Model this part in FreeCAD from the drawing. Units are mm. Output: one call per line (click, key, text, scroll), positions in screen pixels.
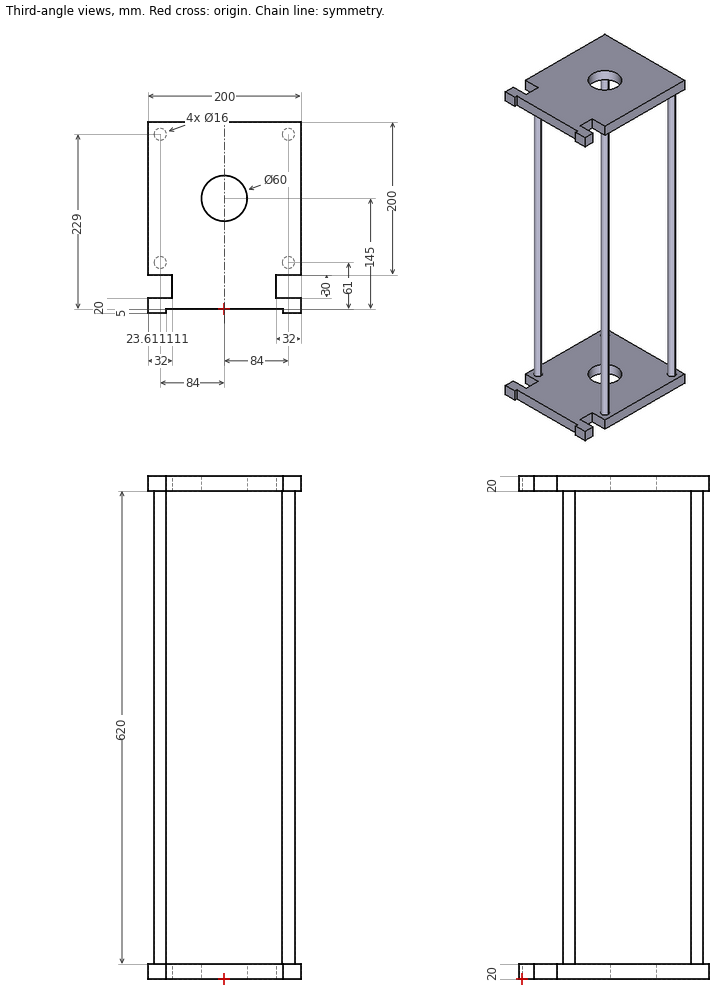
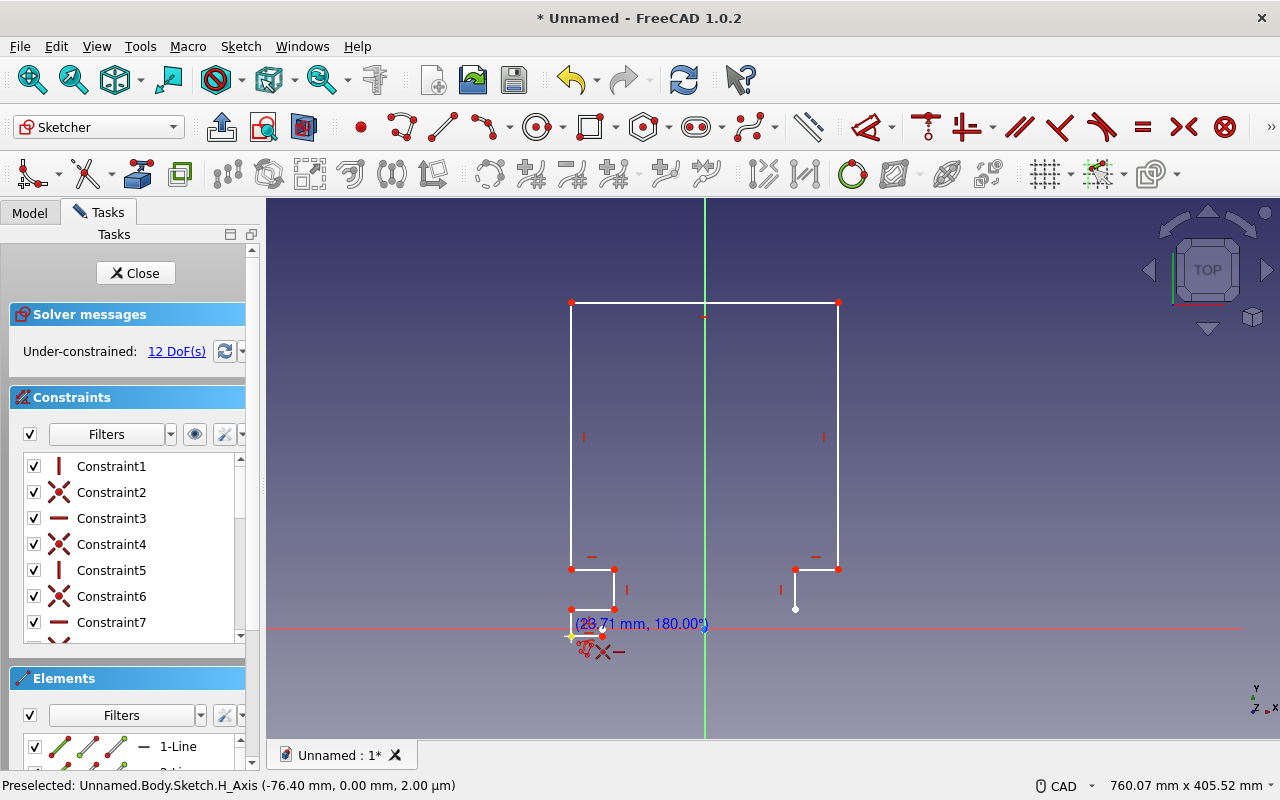
click(807, 620)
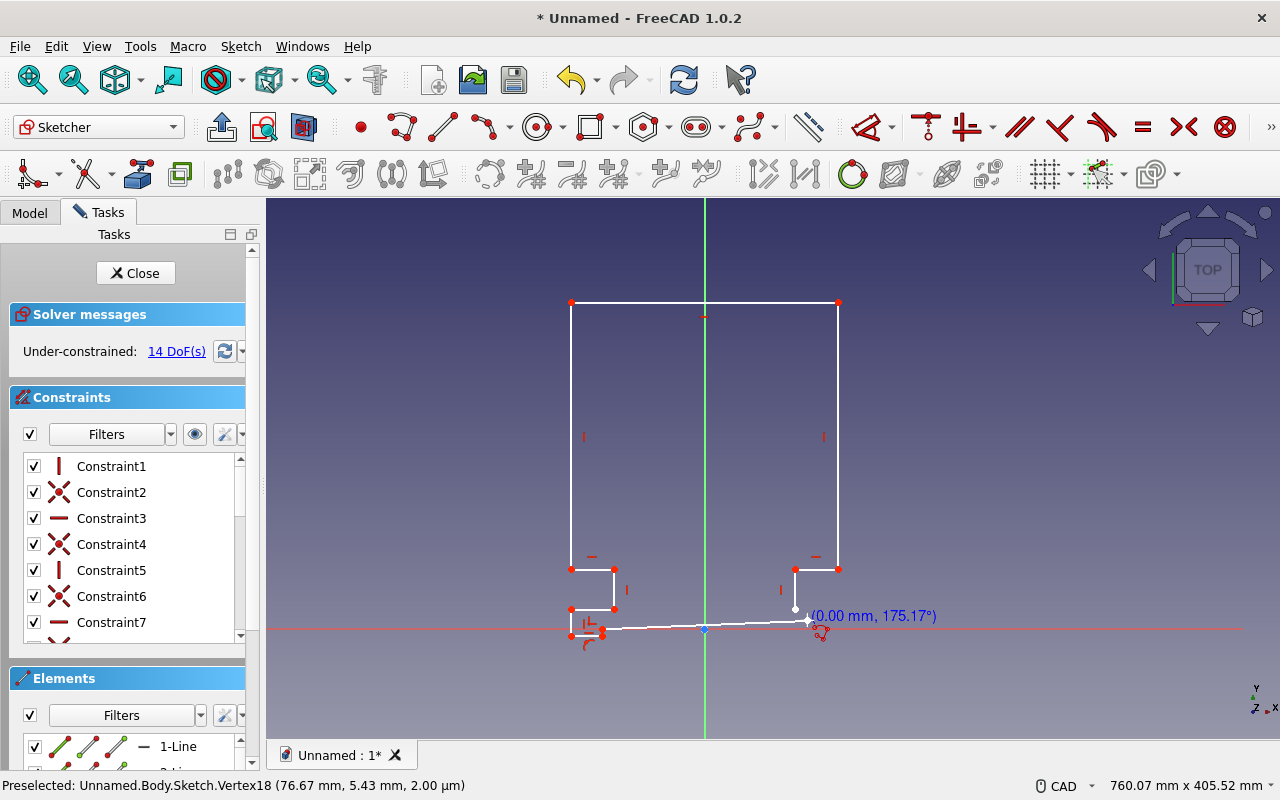
scroll(807, 636, up, 5)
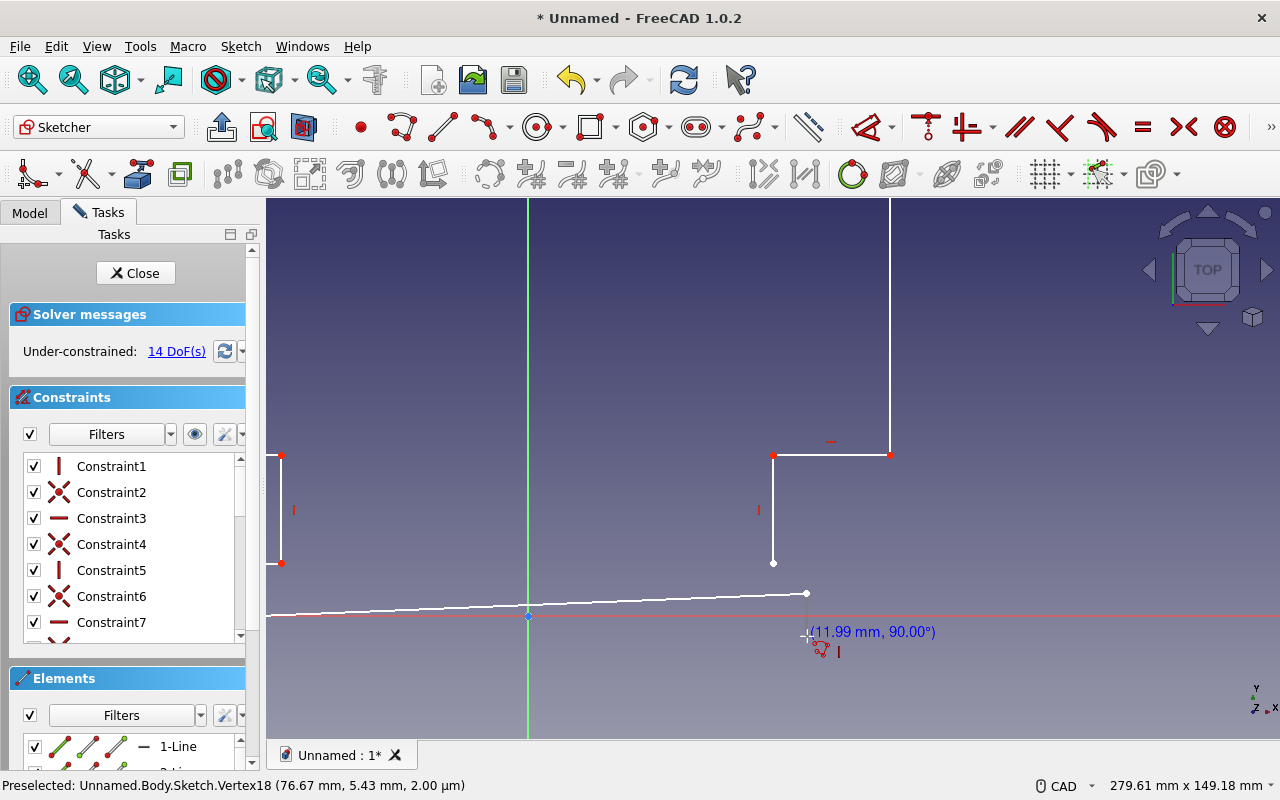
click(806, 634)
click(891, 634)
click(891, 562)
click(773, 564)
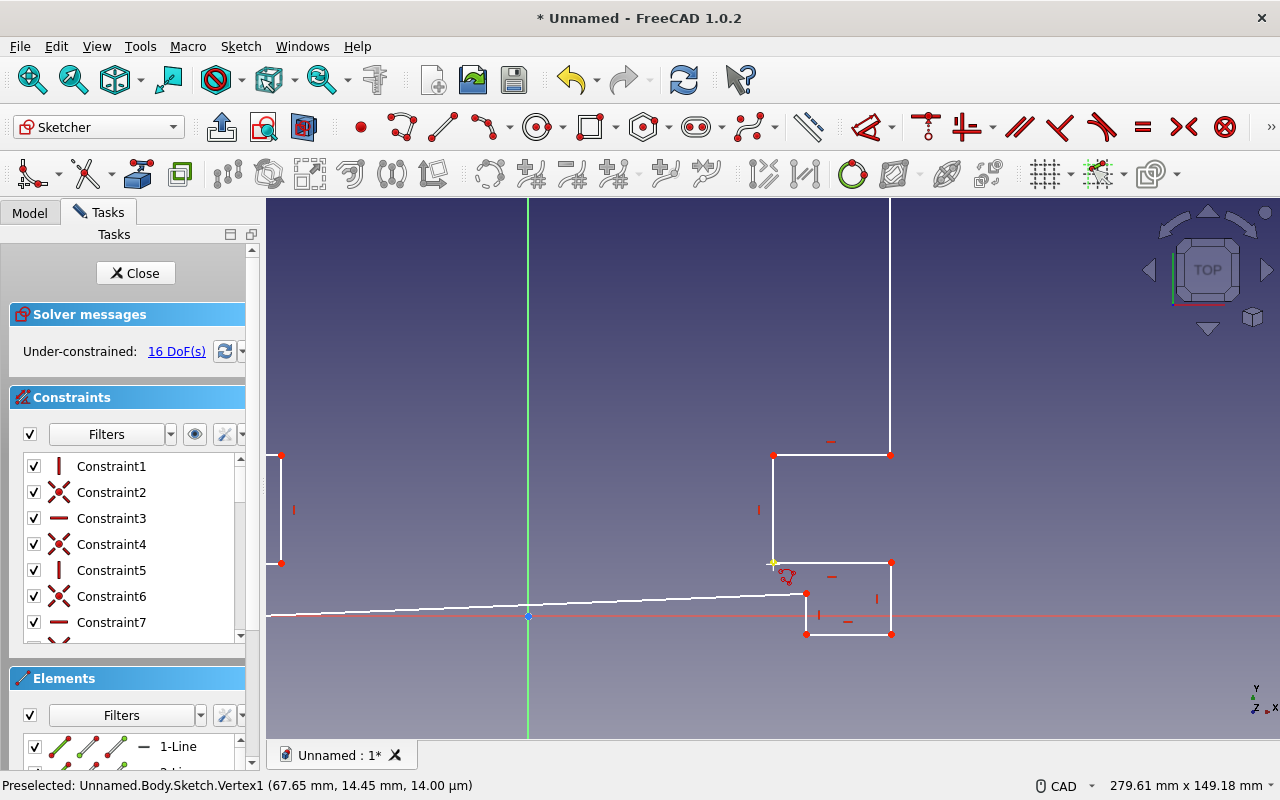
click(536, 128)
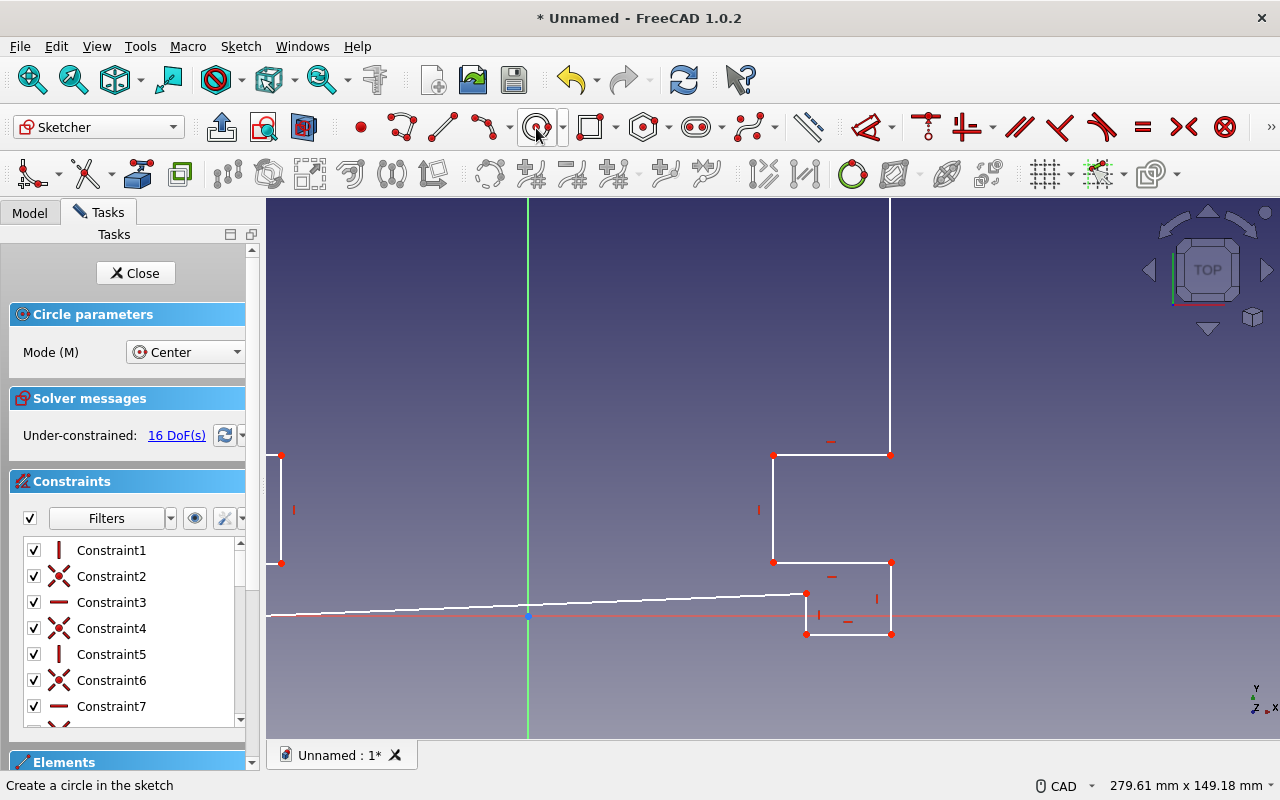
scroll(807, 636, down, 5)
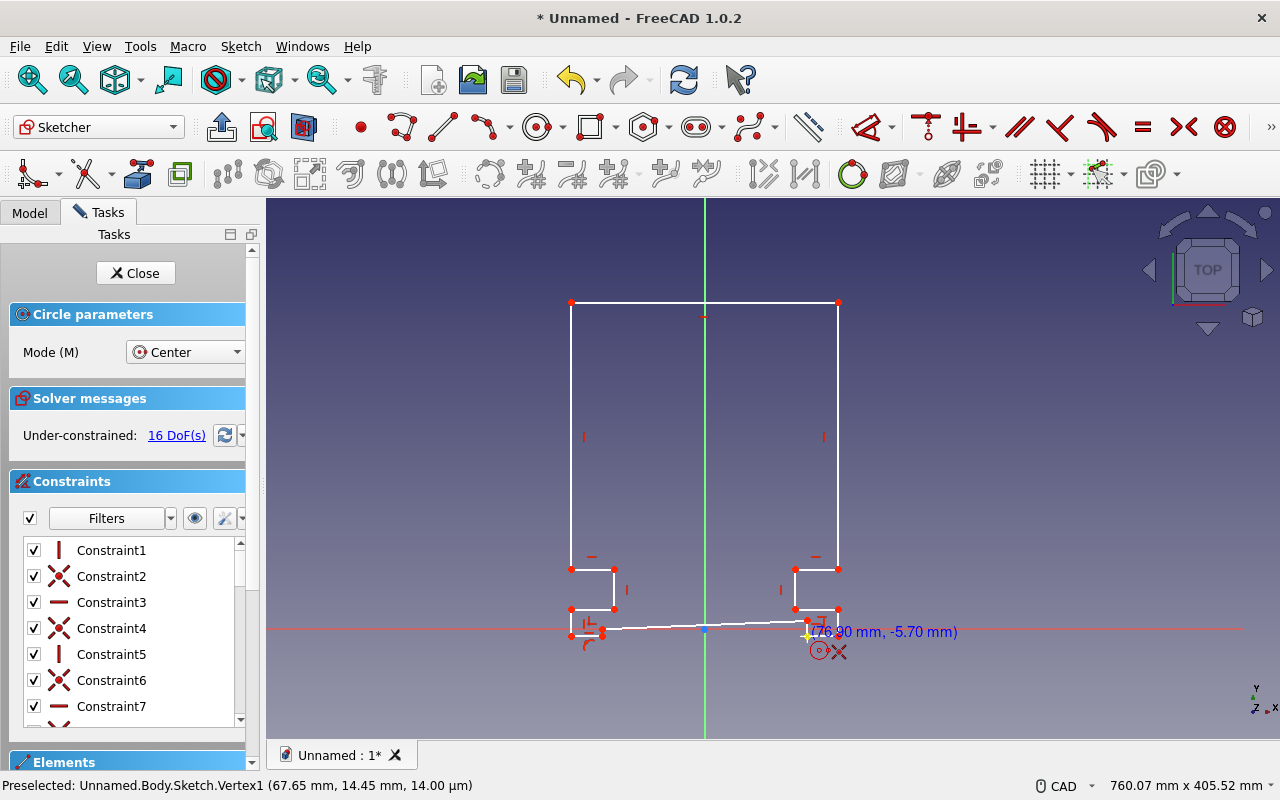
click(705, 436)
click(733, 408)
key(Escape)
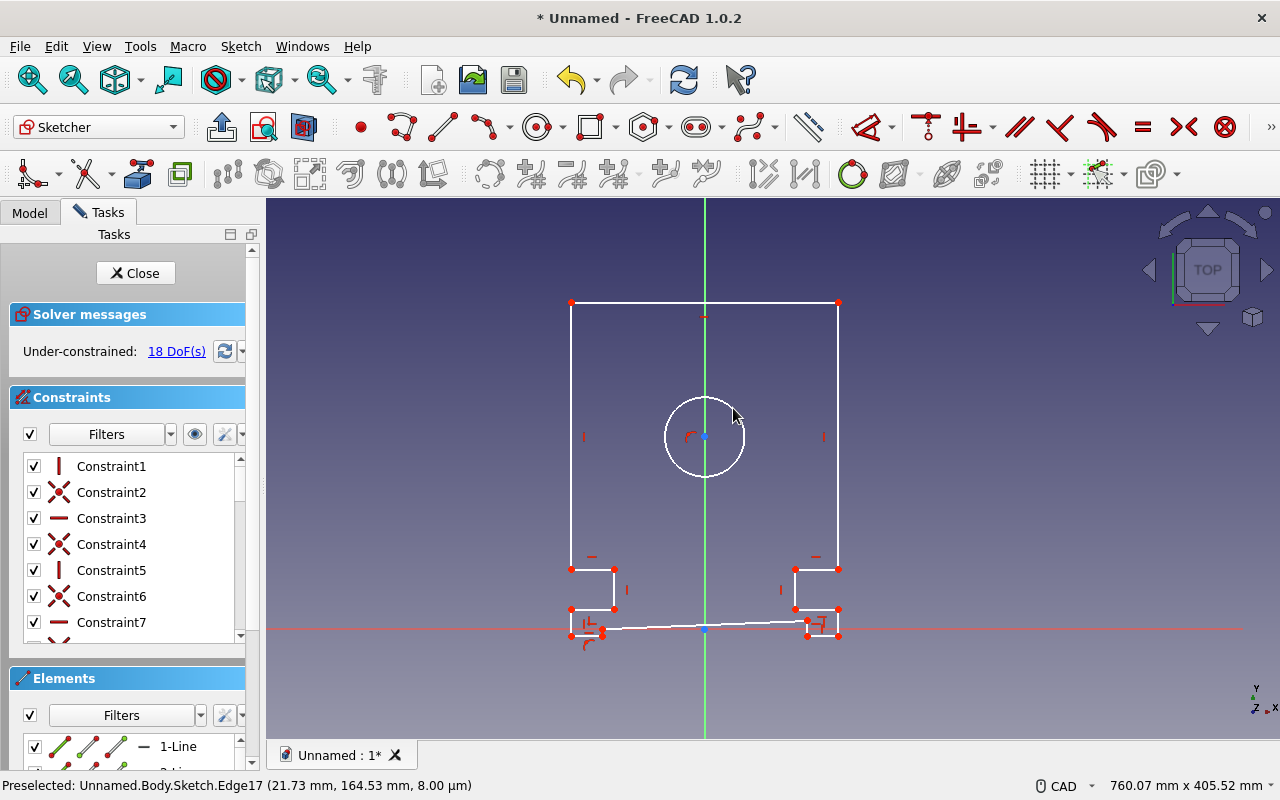
click(664, 627)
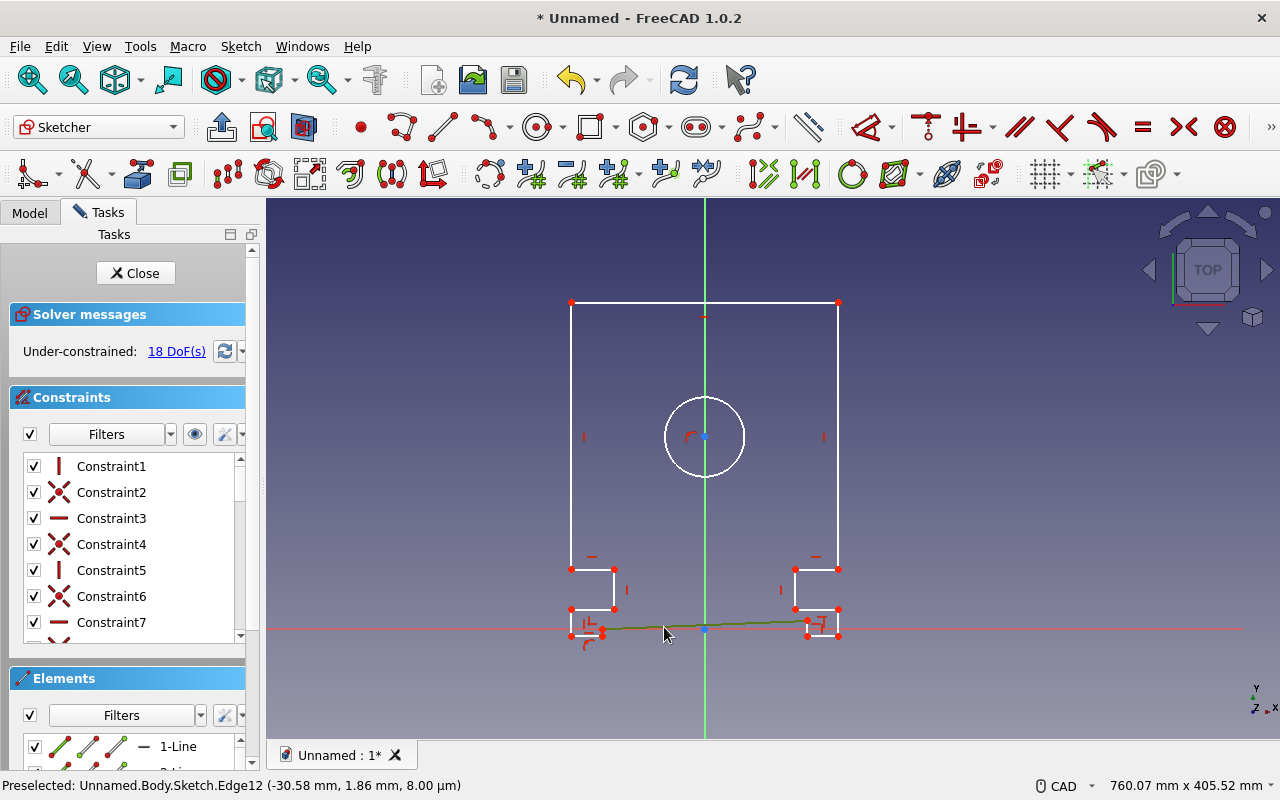
key(h)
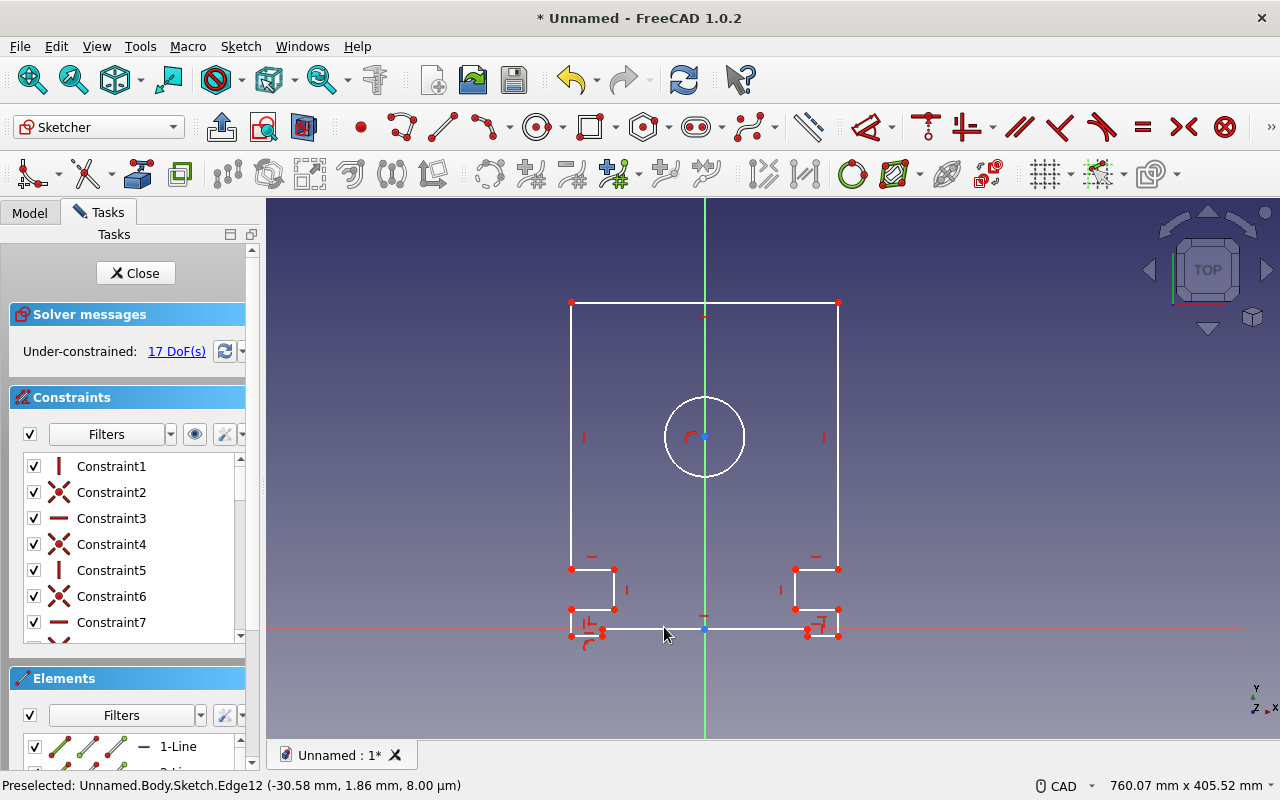
click(838, 570)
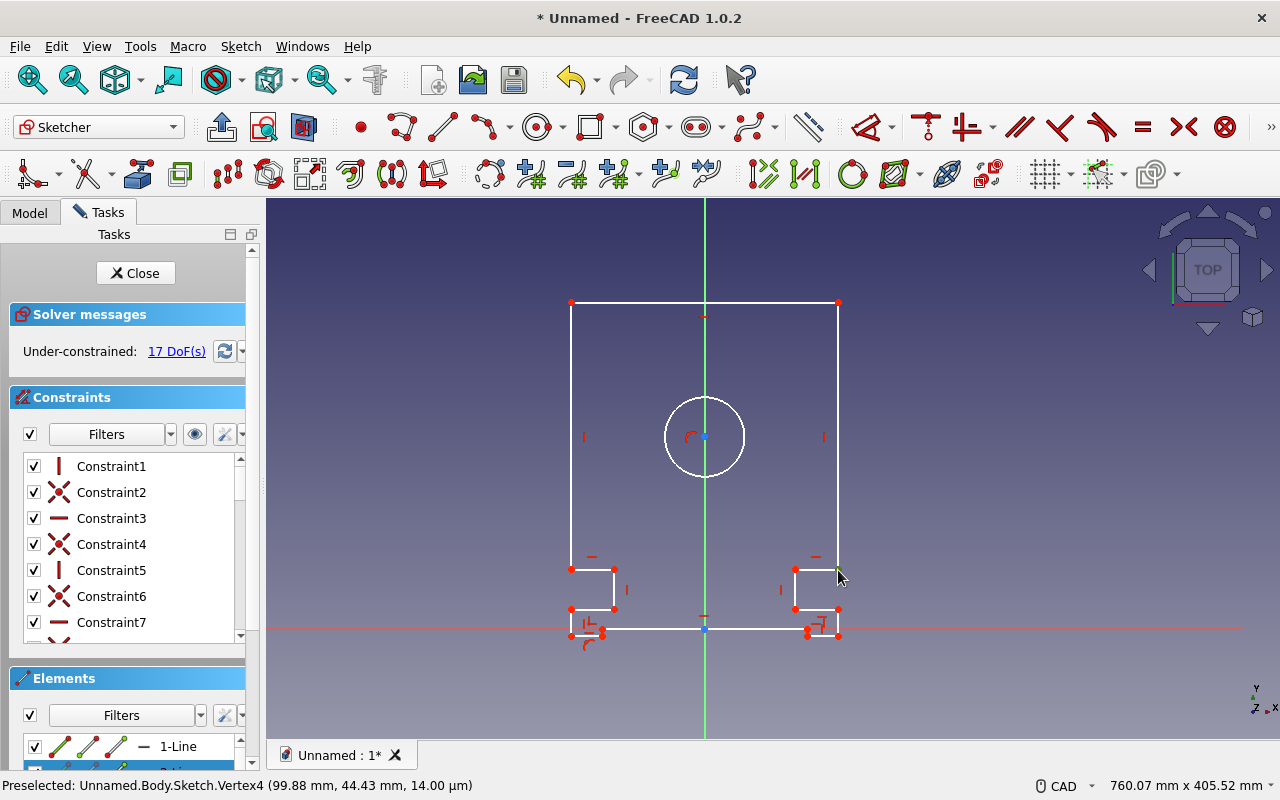
click(571, 570)